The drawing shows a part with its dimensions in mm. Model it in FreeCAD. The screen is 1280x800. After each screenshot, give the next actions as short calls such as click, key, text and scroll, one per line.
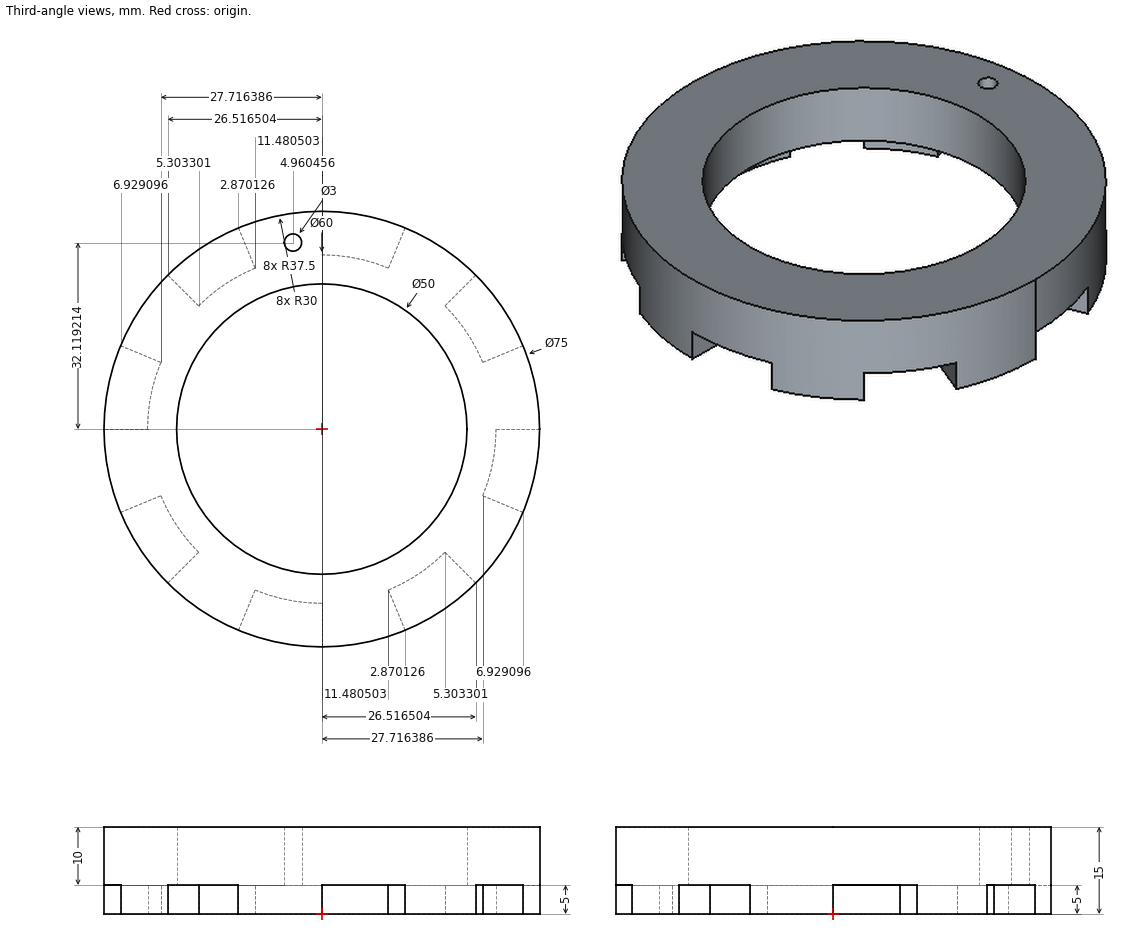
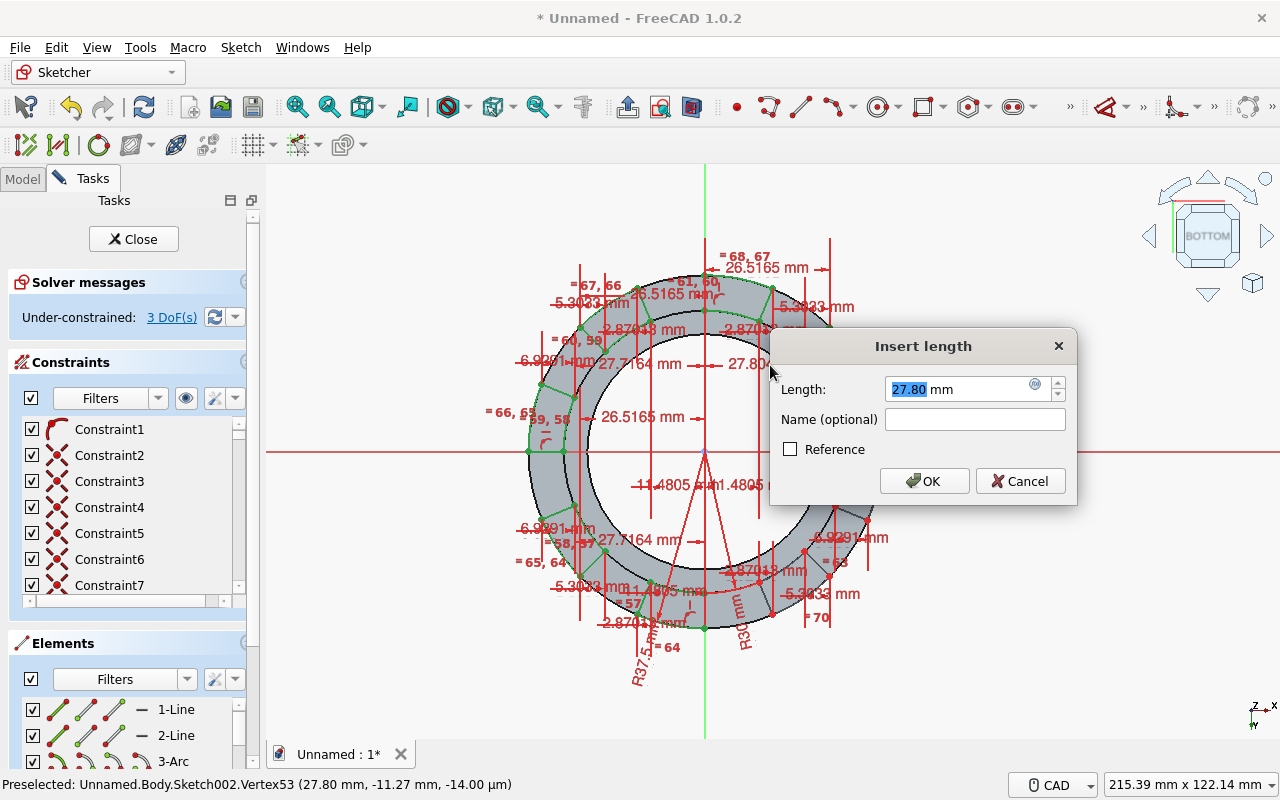
text(27.716386)
key(Return)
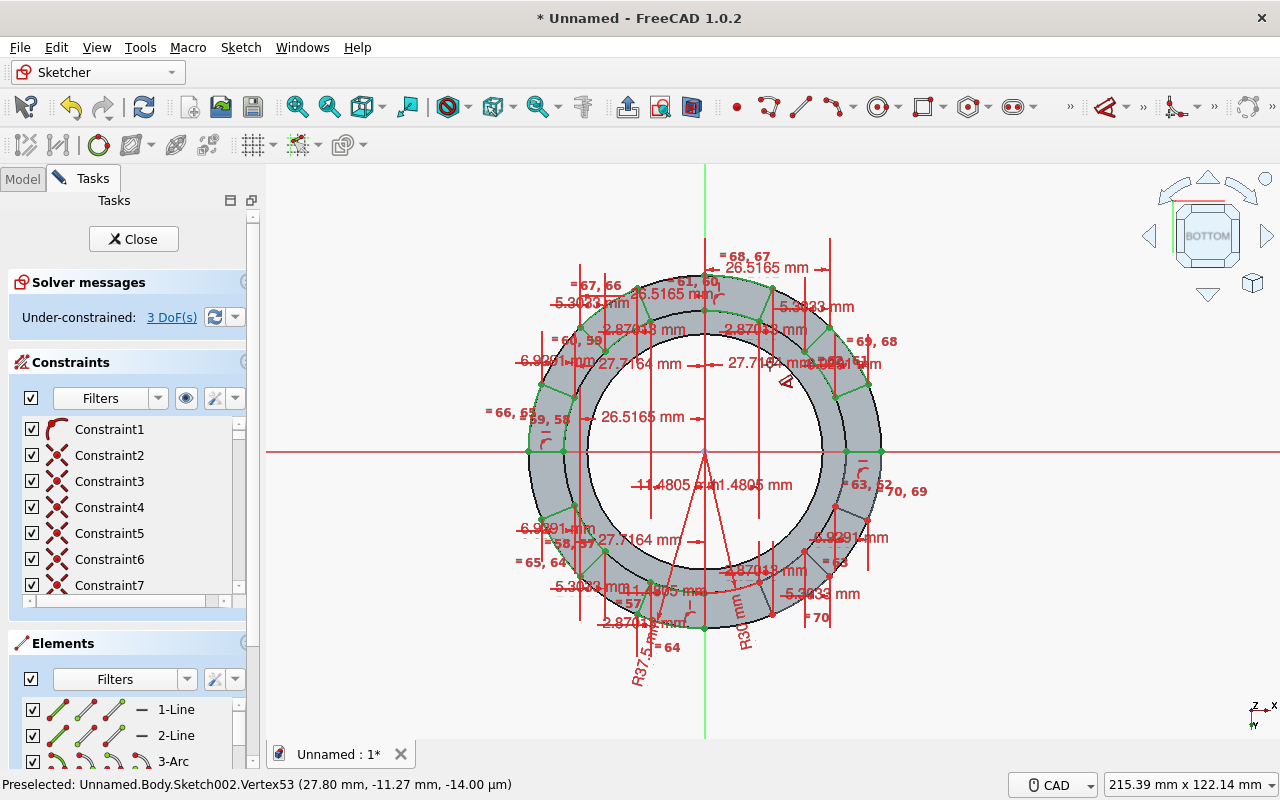
click(835, 507)
click(770, 541)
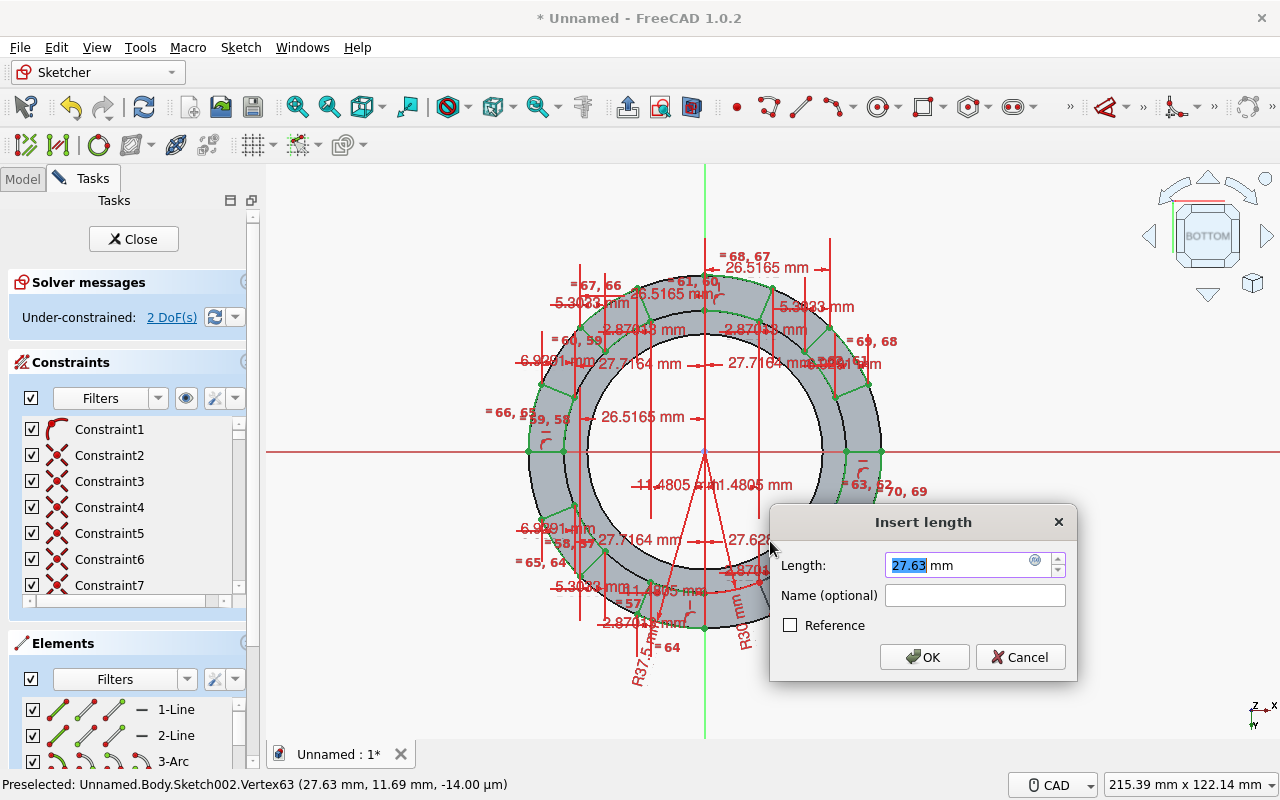
text(27.716386)
key(Return)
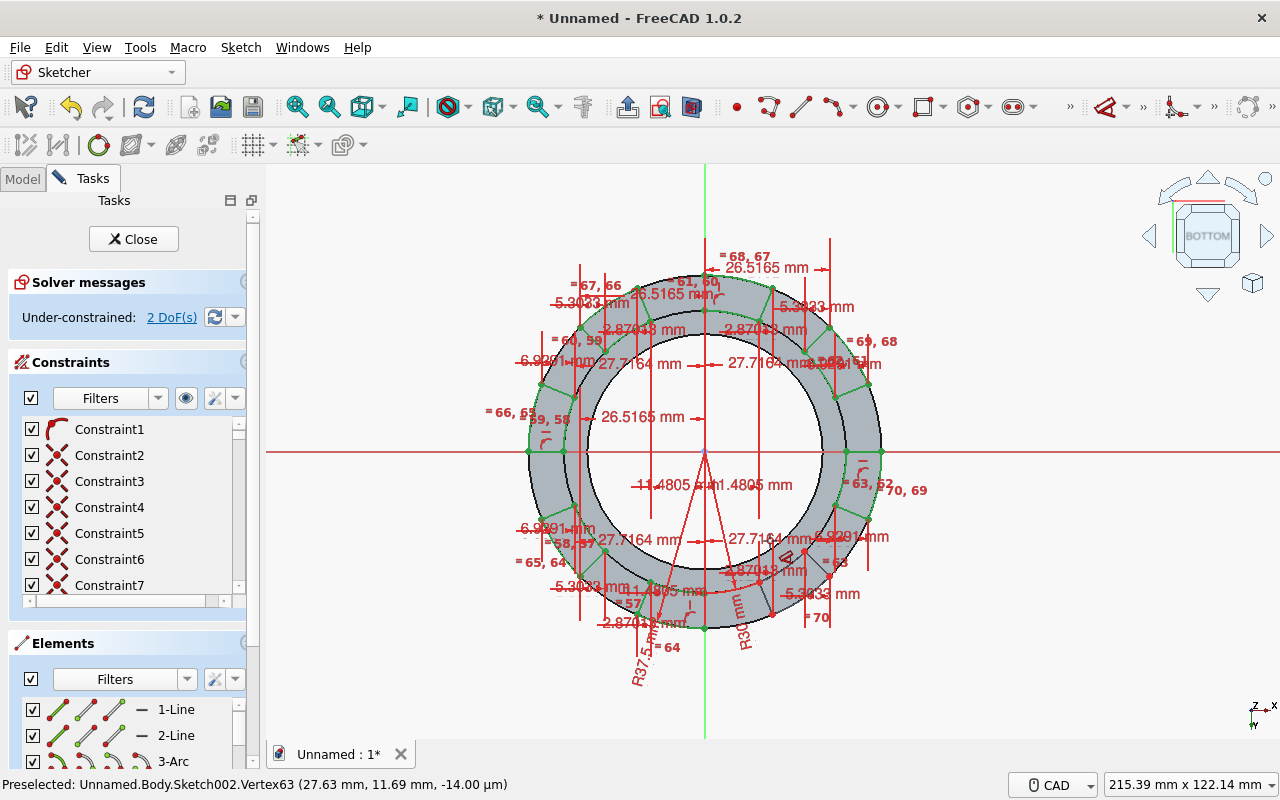
click(830, 577)
click(767, 418)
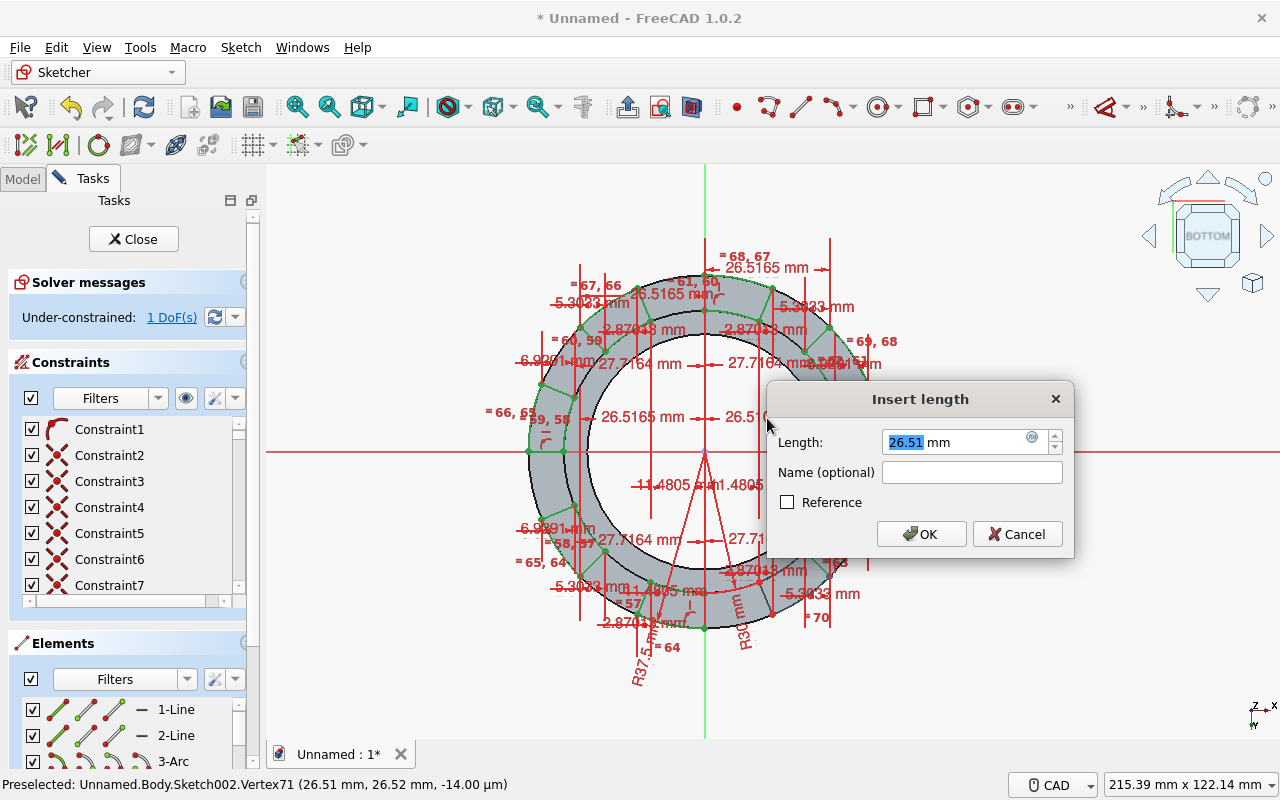
text(26.516504)
key(Return)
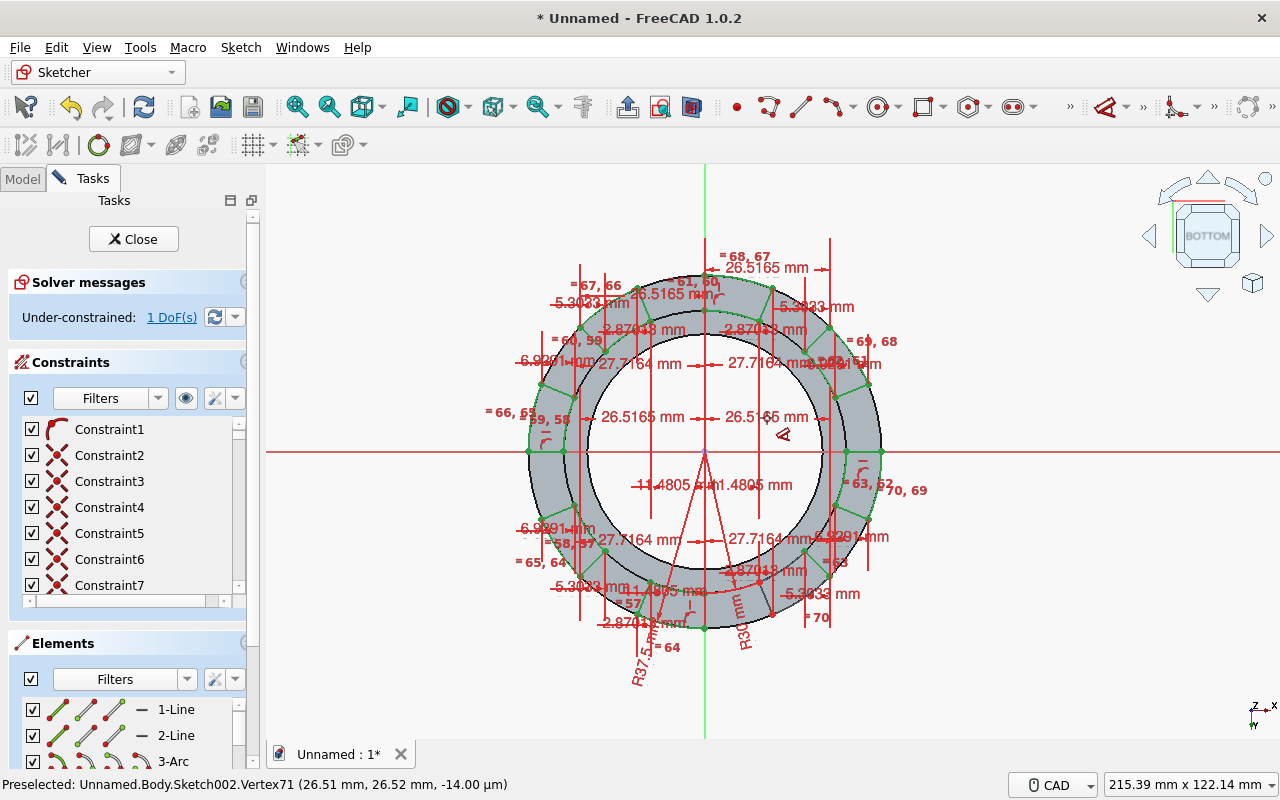
click(759, 582)
click(732, 394)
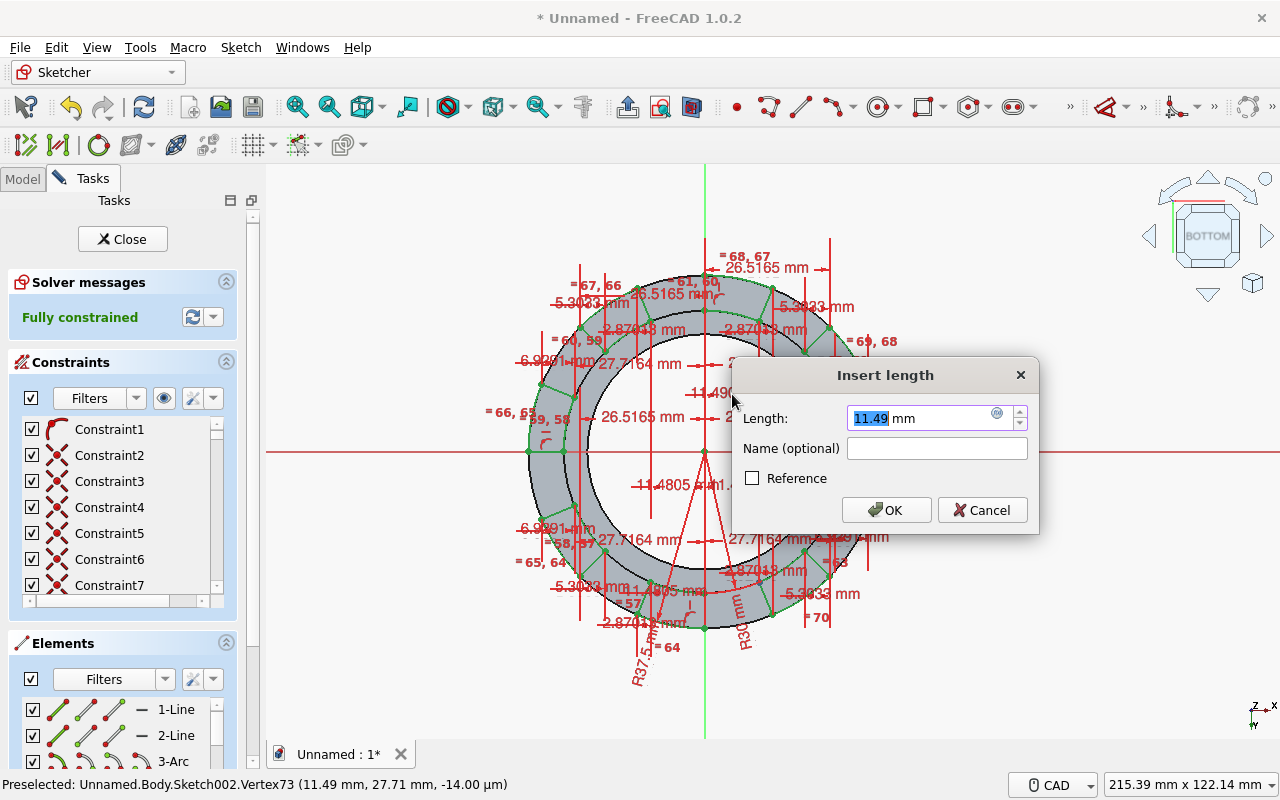
text(11.480503)
key(Return)
key(Escape)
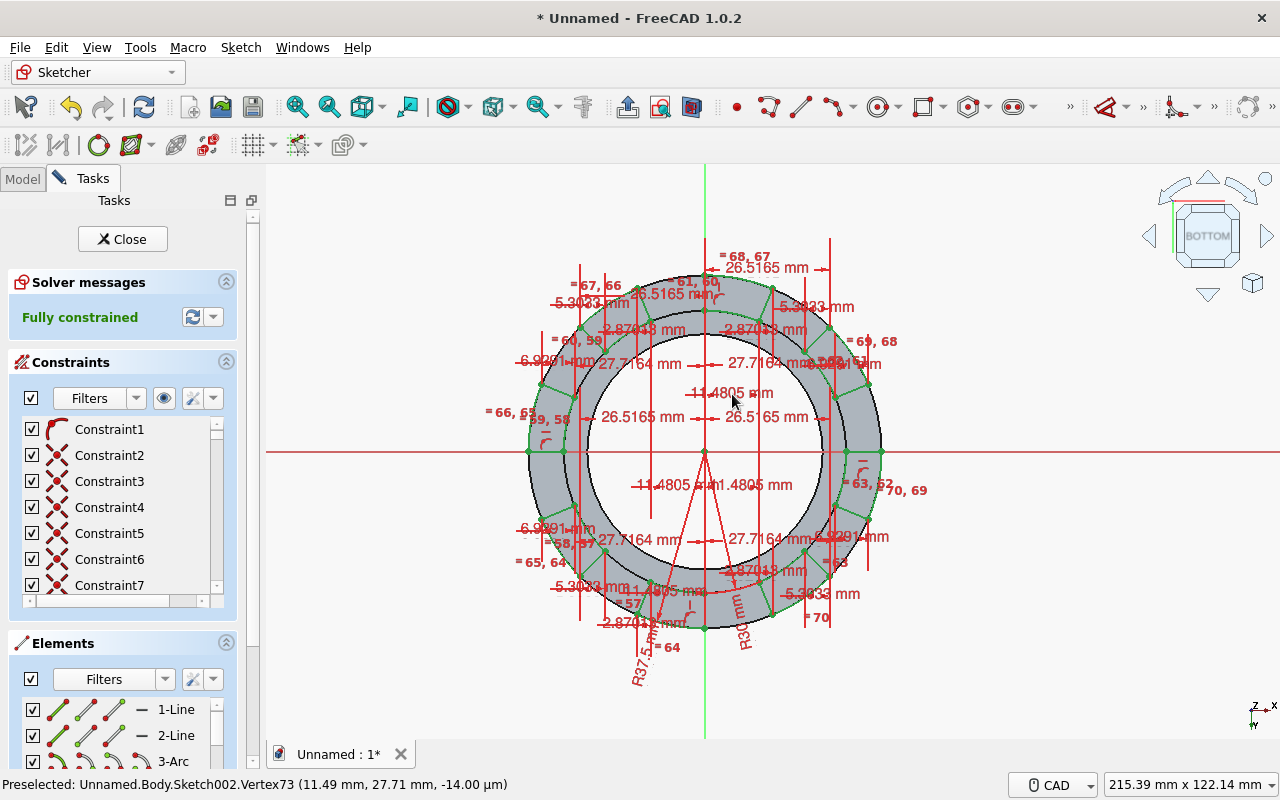
click(123, 239)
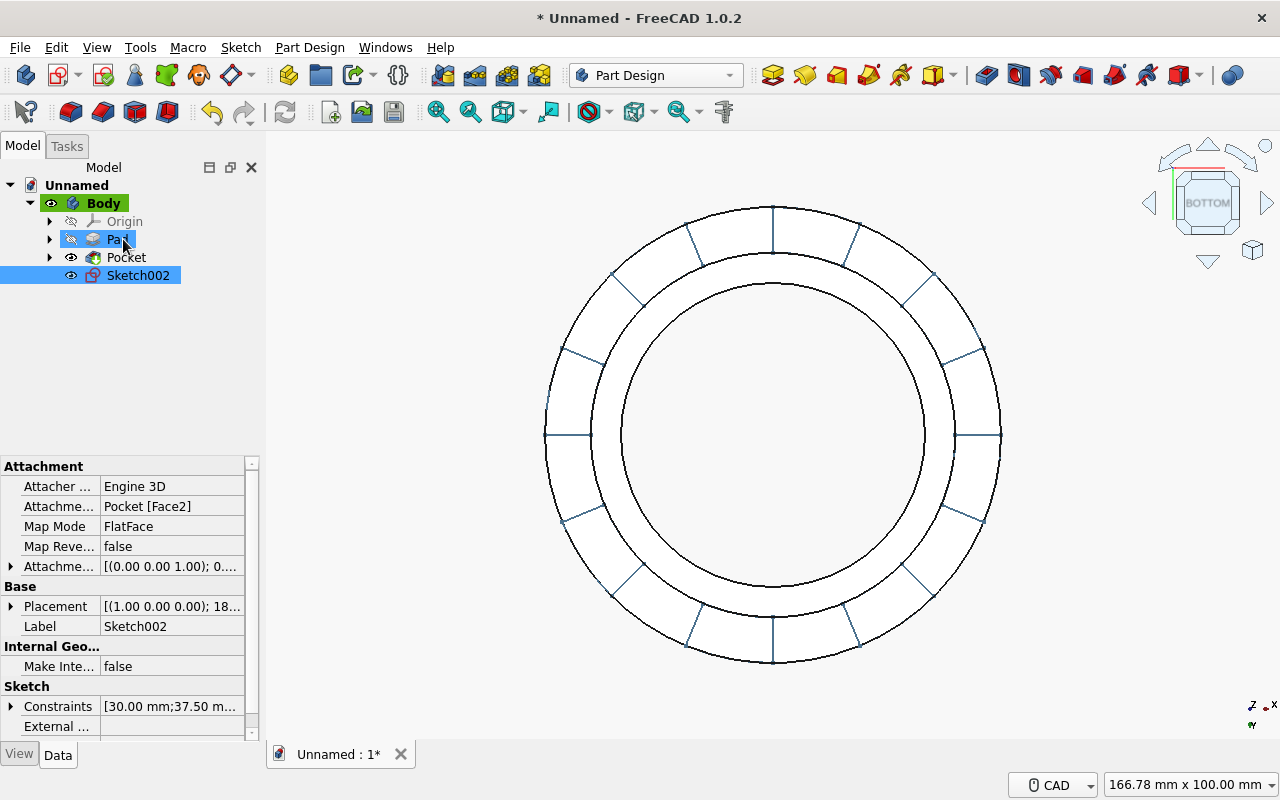
click(988, 76)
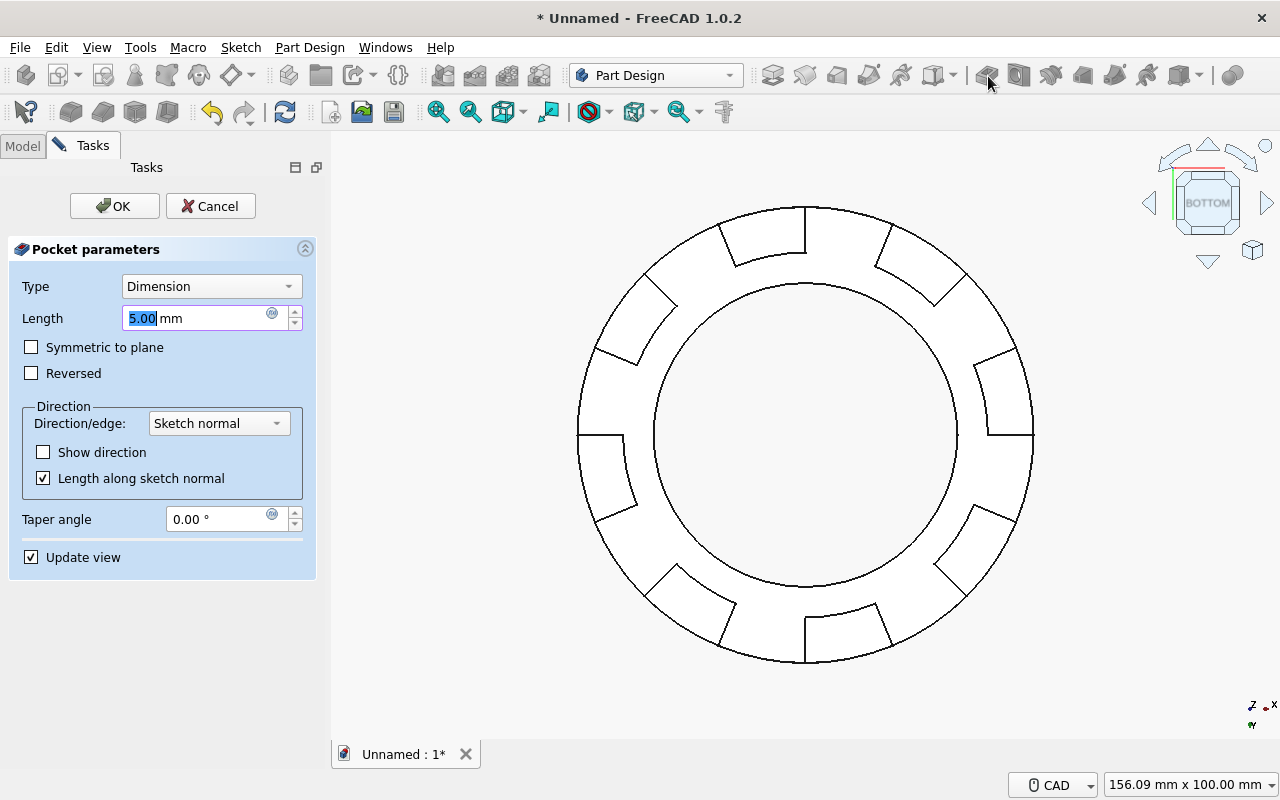
text(5)
key(Tab)